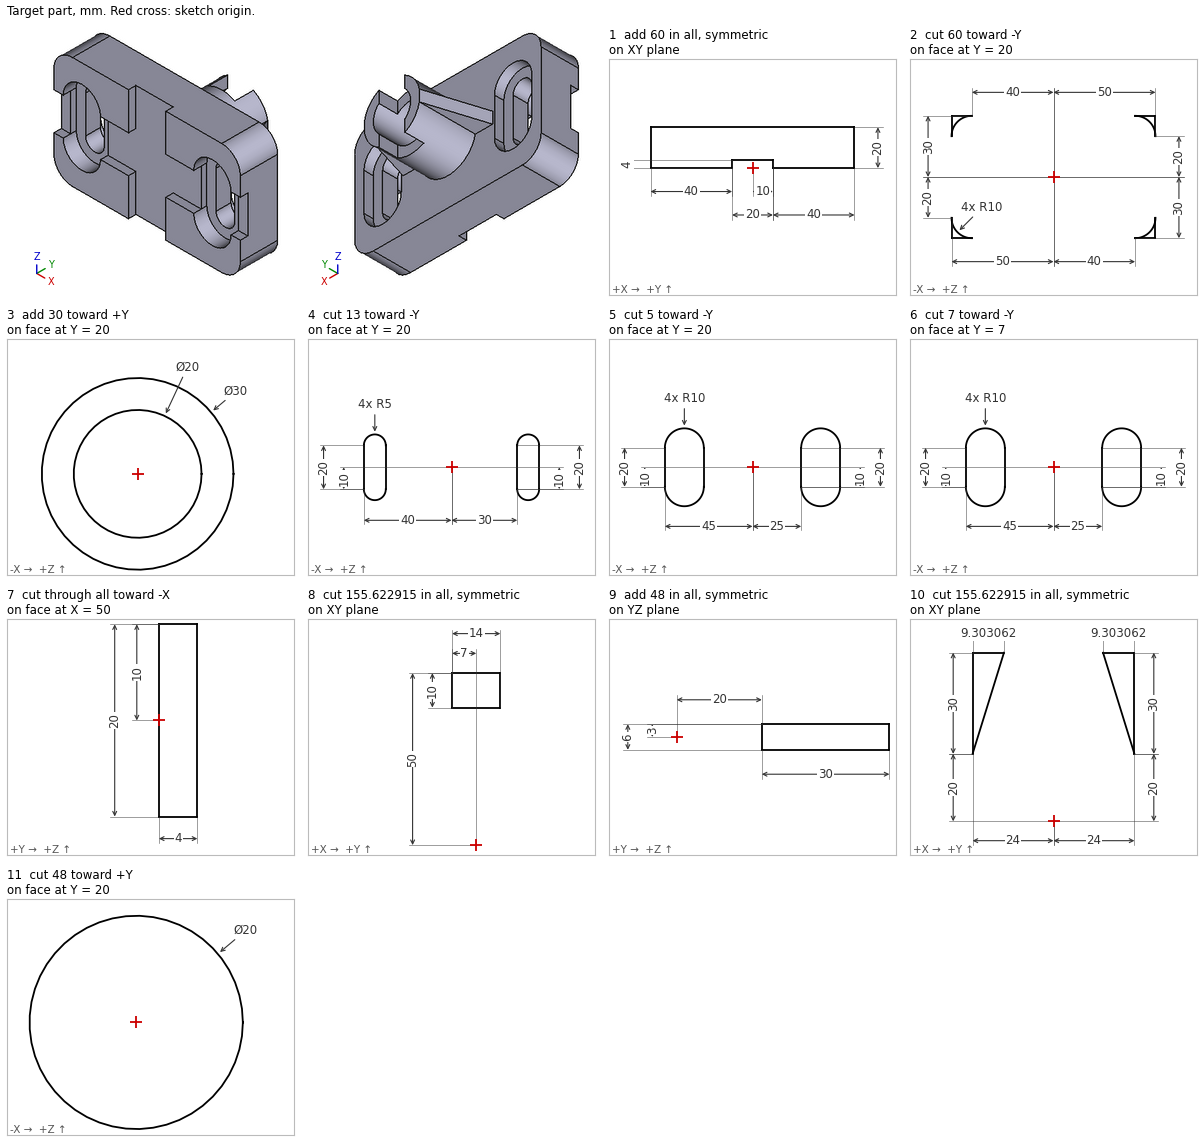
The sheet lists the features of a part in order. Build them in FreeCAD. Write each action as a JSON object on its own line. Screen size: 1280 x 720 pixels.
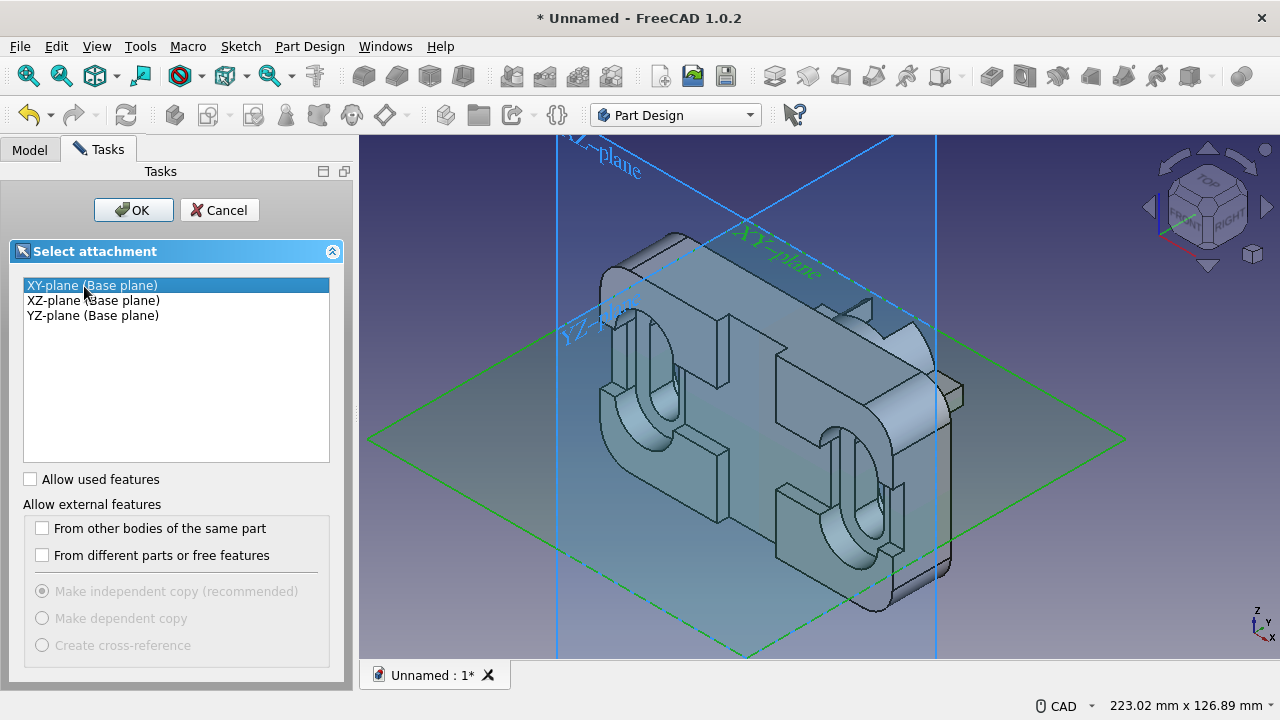
{"action": "left_click", "coordinate": [134, 210]}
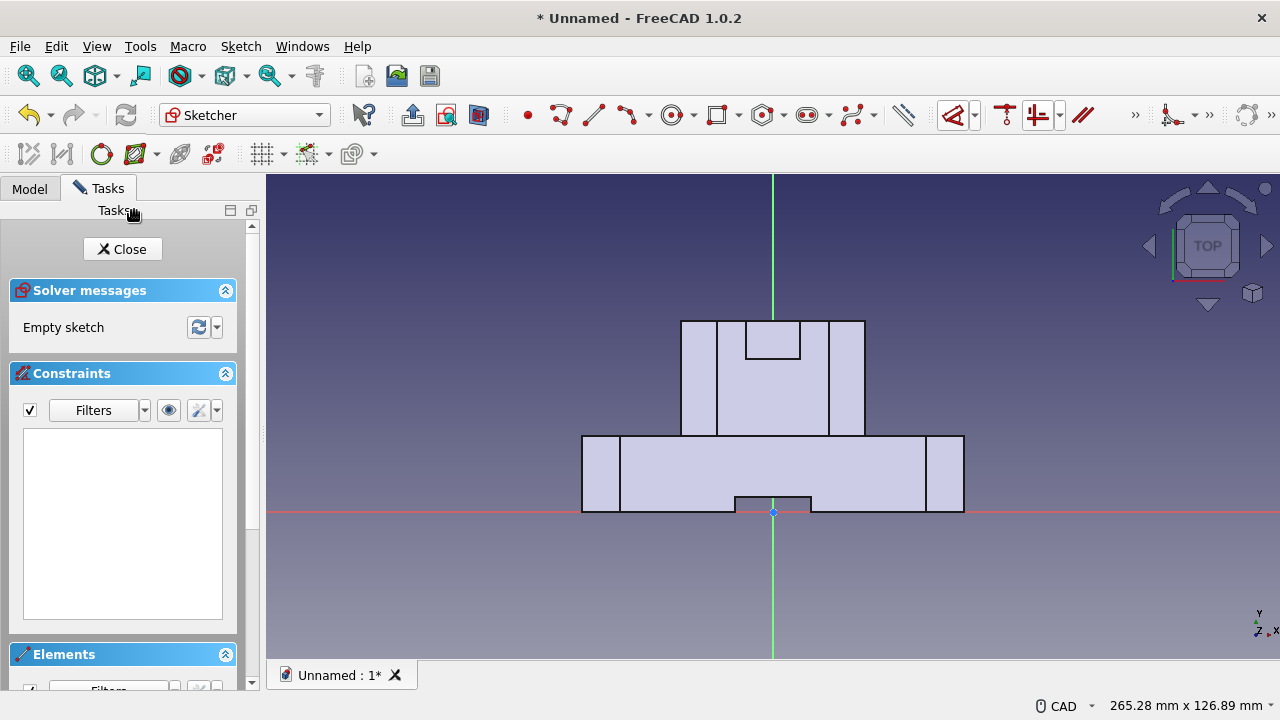
{"action": "key", "text": "q s"}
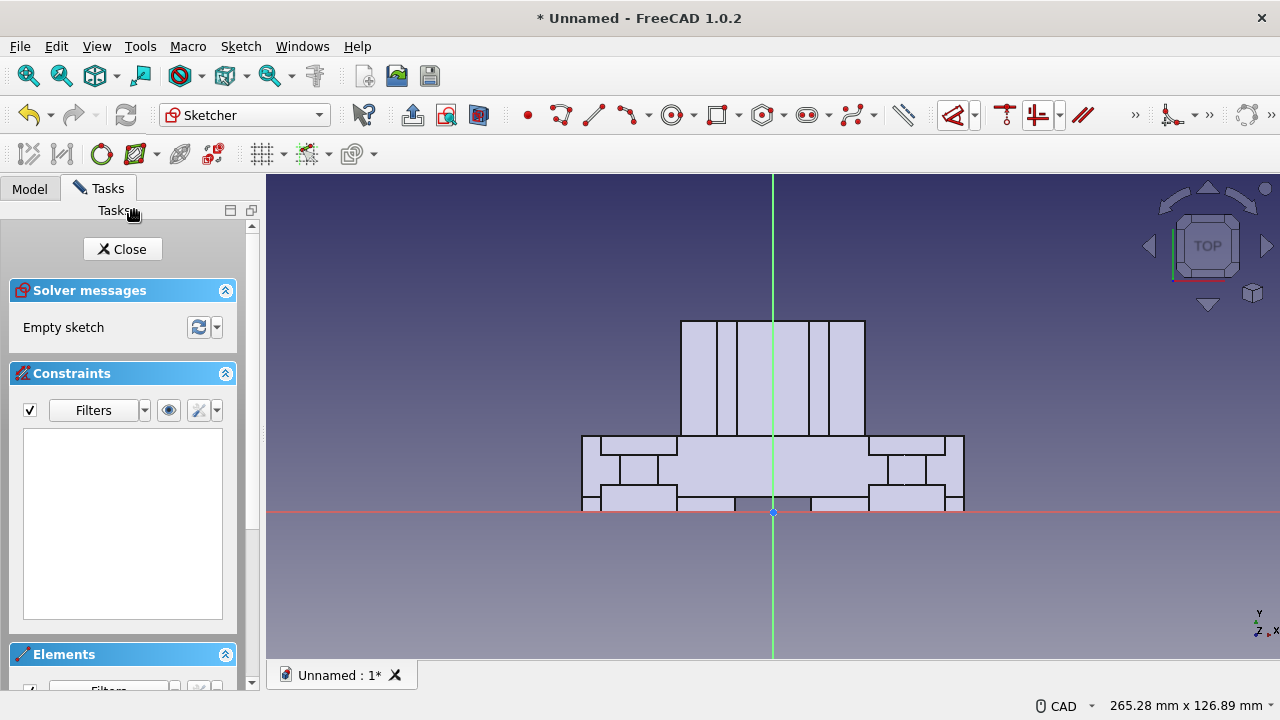
{"action": "scroll", "coordinate": [912, 416], "scroll_direction": "up", "scroll_amount": 2}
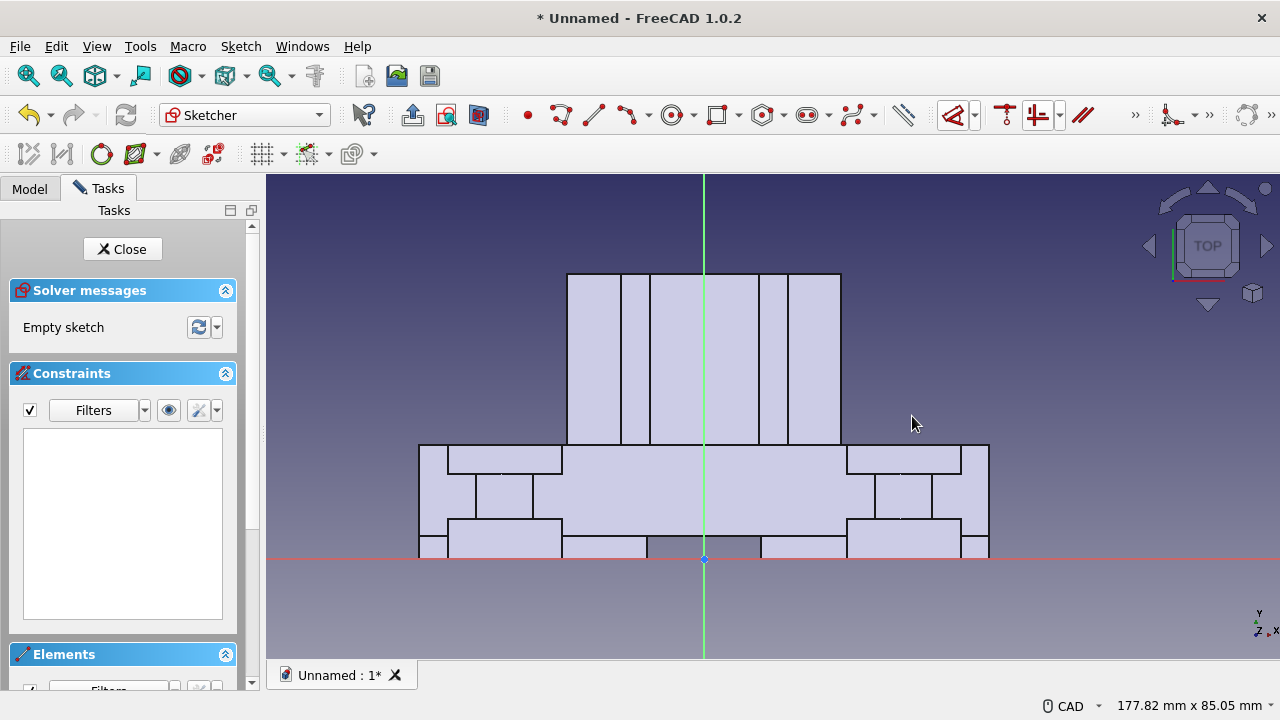
{"action": "left_click", "coordinate": [561, 116]}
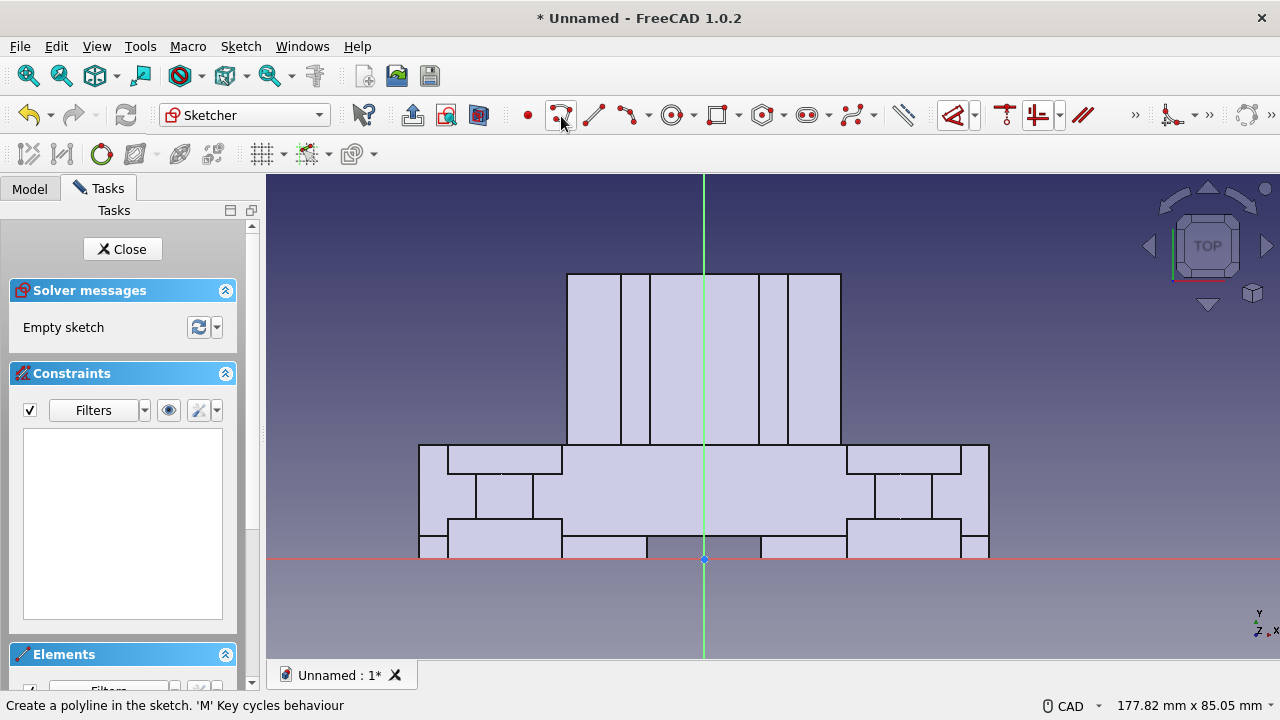
{"action": "left_click", "coordinate": [841, 445]}
{"action": "left_click", "coordinate": [841, 274]}
{"action": "left_click", "coordinate": [788, 274]}
{"action": "left_click", "coordinate": [841, 446]}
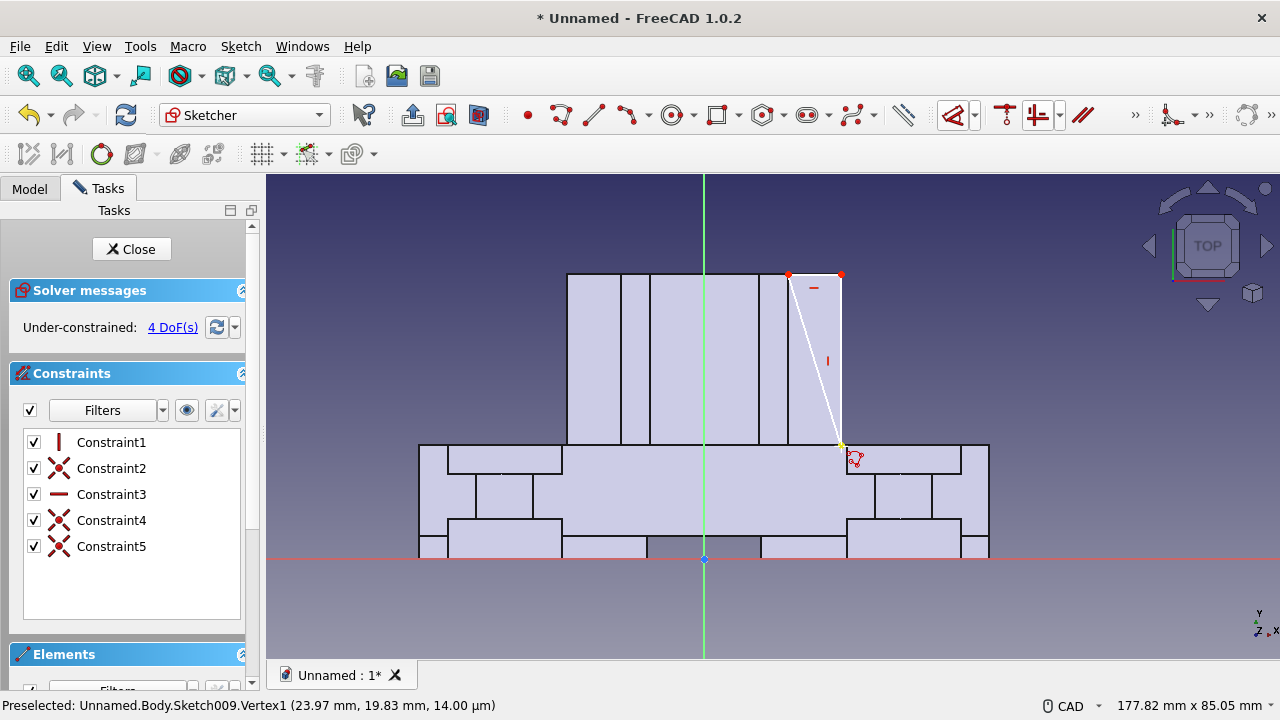
{"action": "left_click", "coordinate": [567, 445]}
{"action": "left_click", "coordinate": [621, 274]}
{"action": "left_click", "coordinate": [567, 274]}
{"action": "left_click", "coordinate": [567, 446]}
{"action": "key", "text": "Escape"}
{"action": "key", "text": "Escape"}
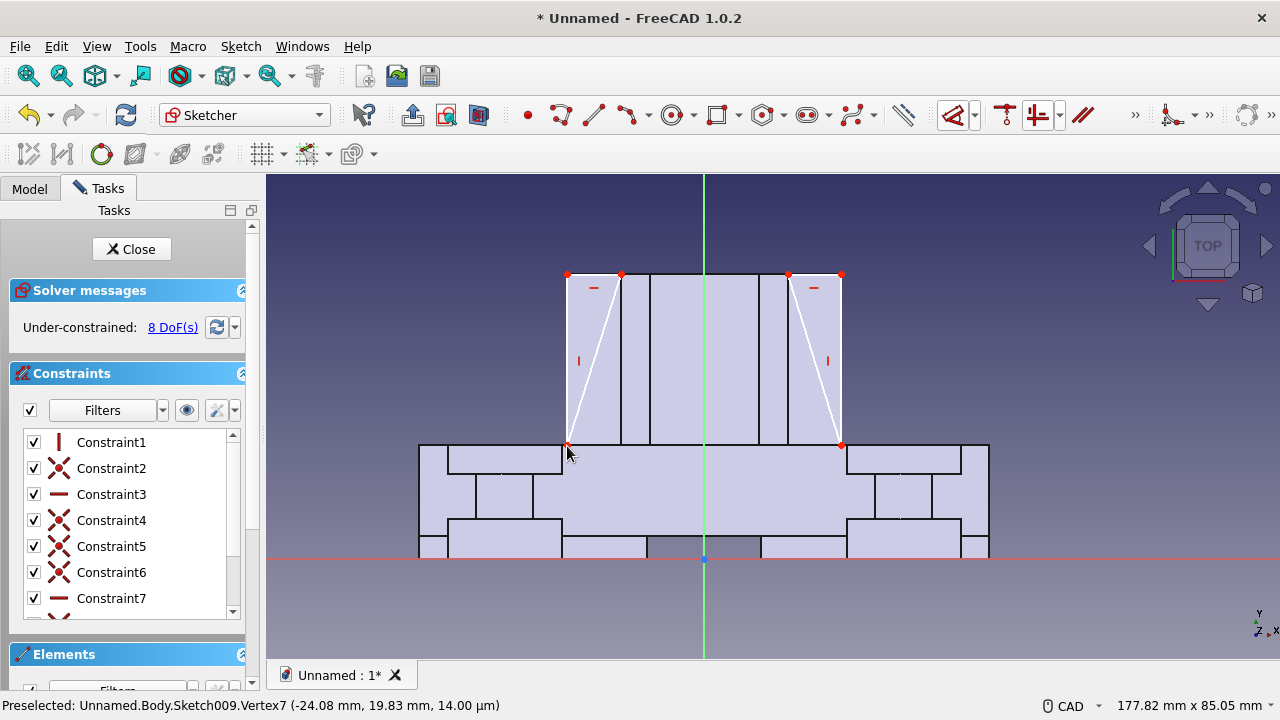
{"action": "left_click", "coordinate": [841, 395]}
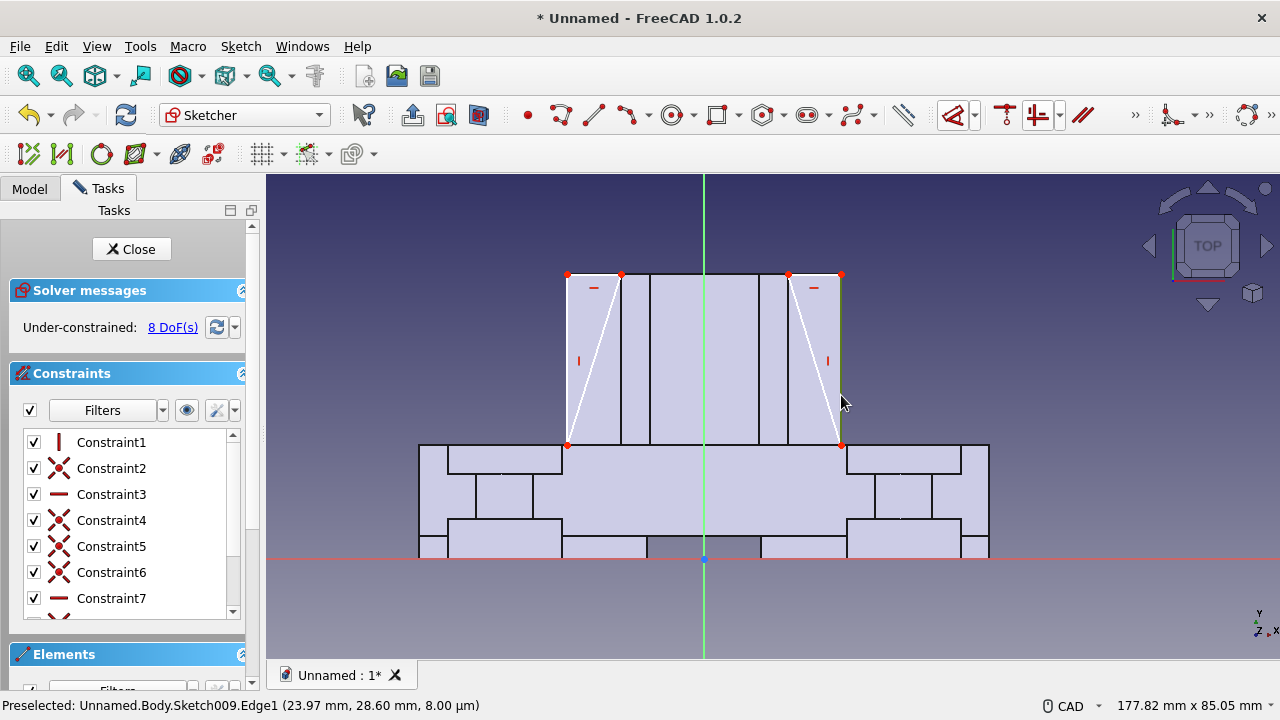
{"action": "key", "text": "i"}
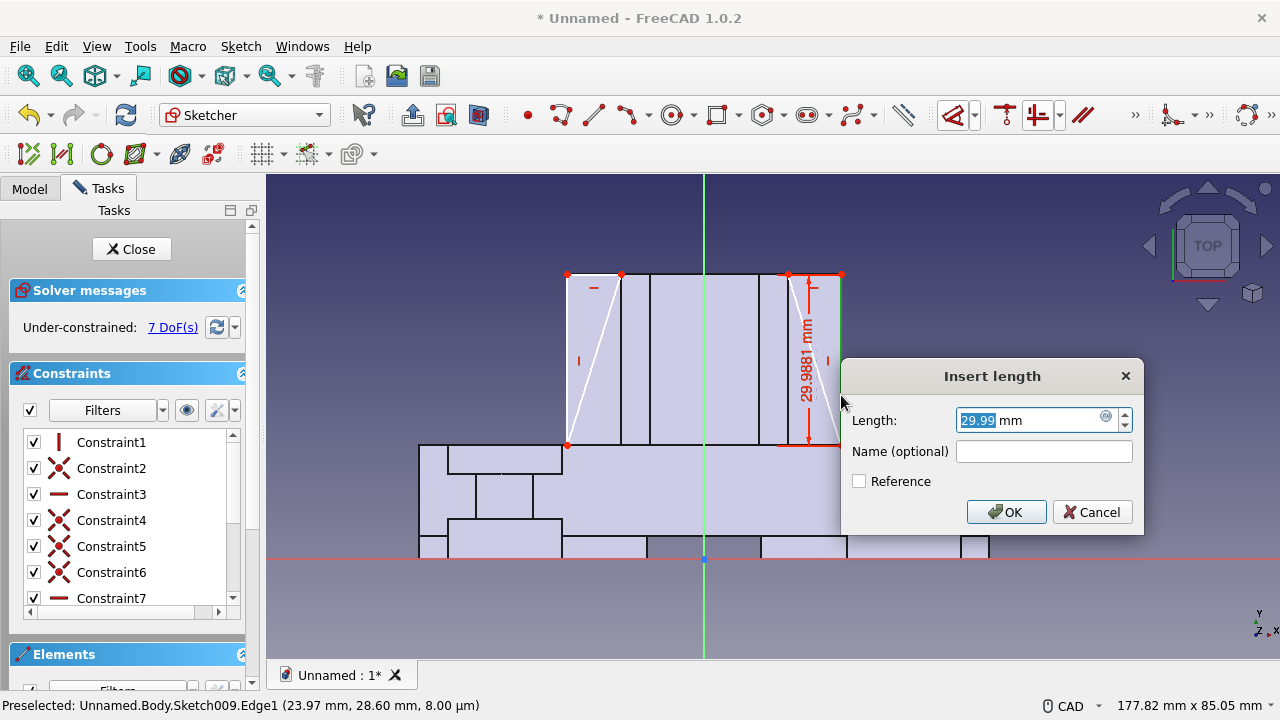
{"action": "type", "text": "30"}
{"action": "key", "text": "Return"}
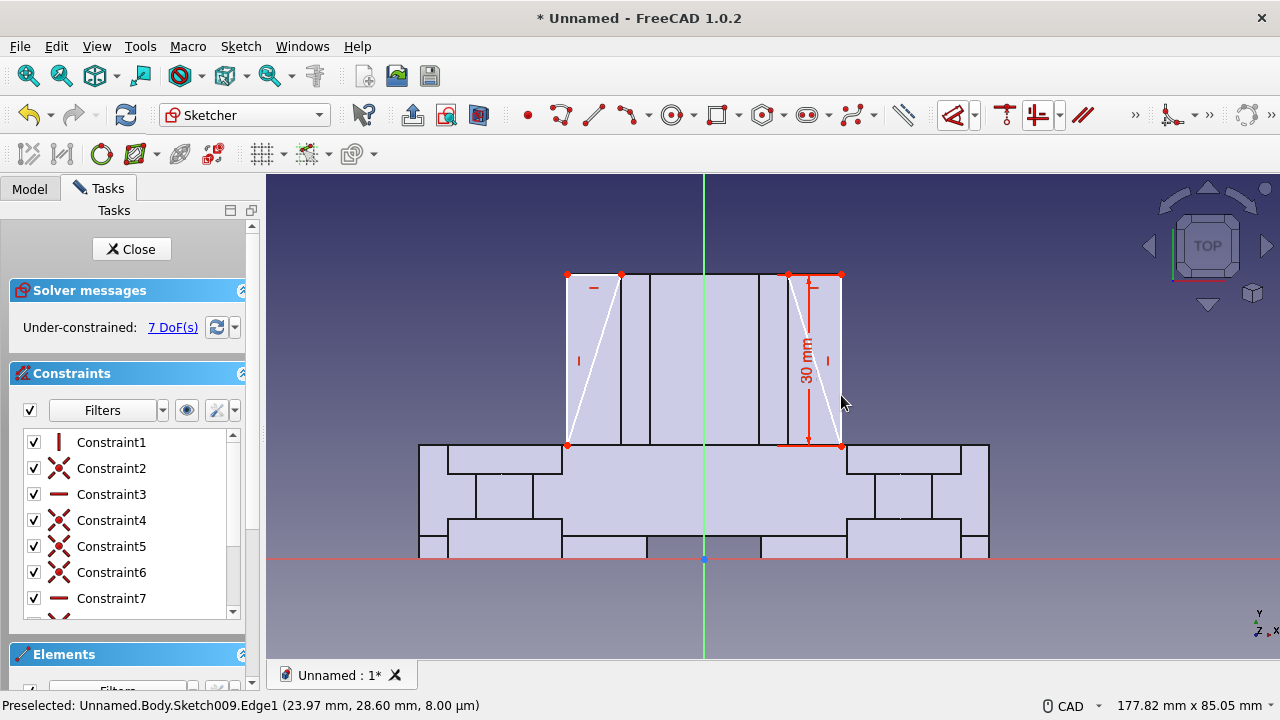
{"action": "left_click", "coordinate": [567, 326]}